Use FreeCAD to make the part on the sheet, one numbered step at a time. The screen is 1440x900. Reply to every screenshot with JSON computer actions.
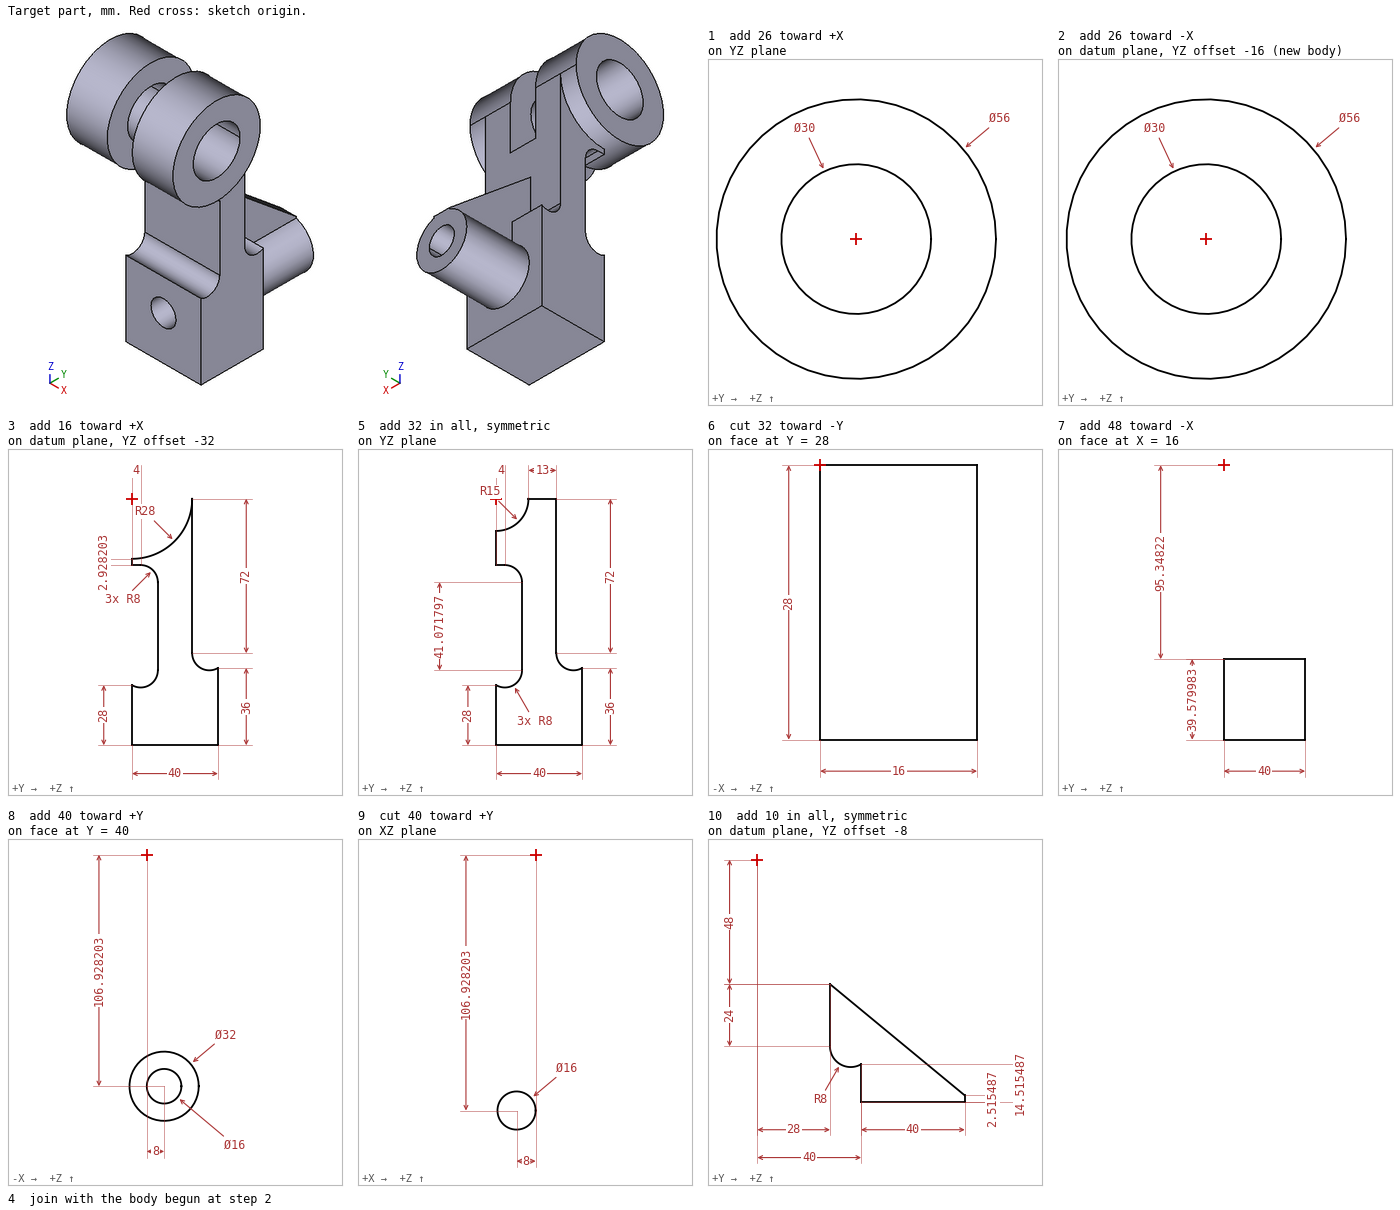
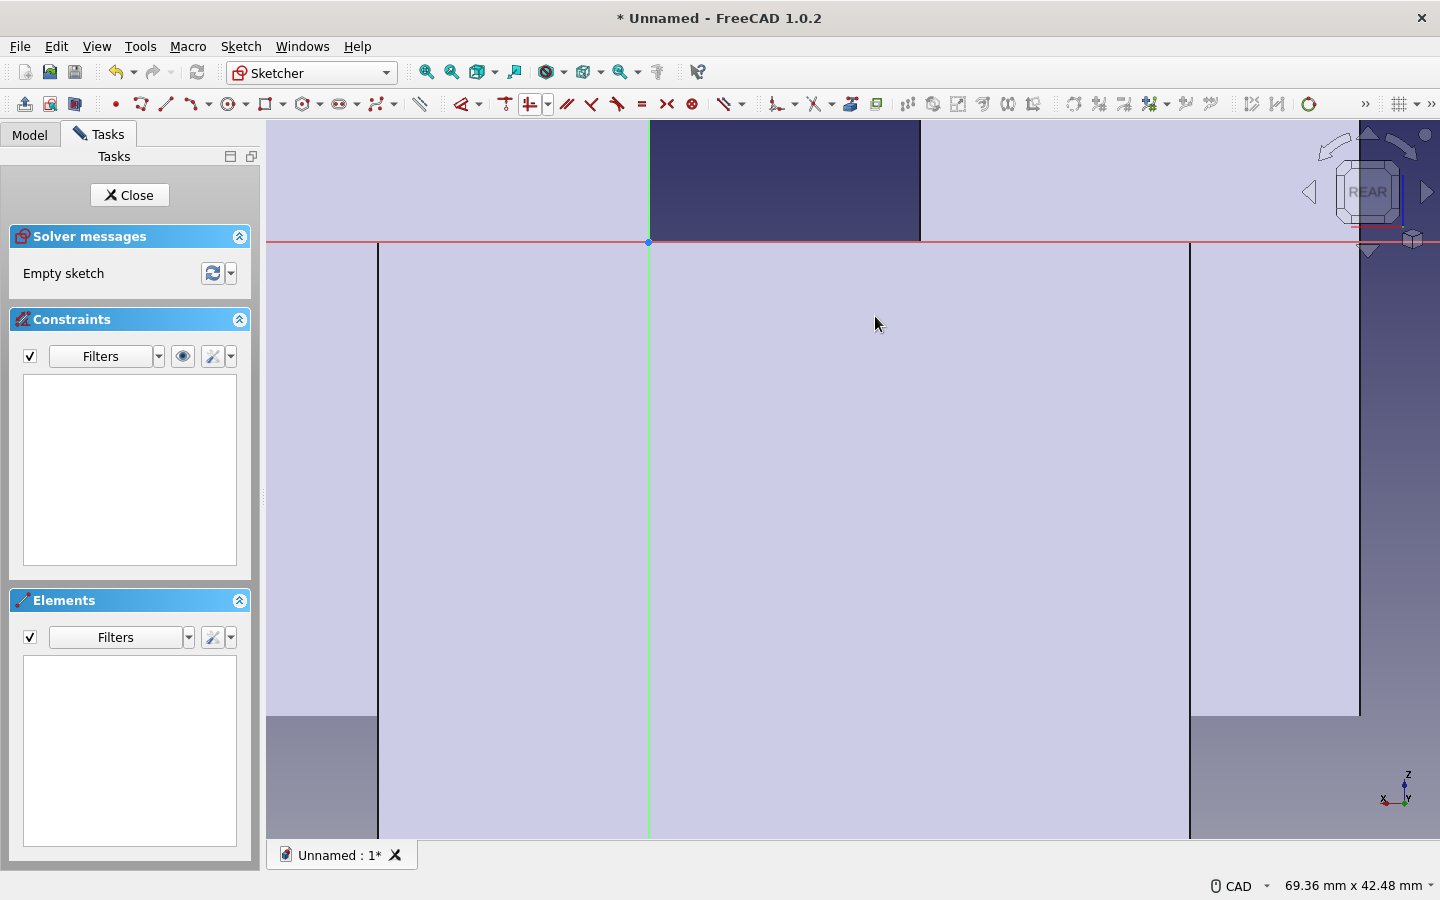
{"action": "key", "text": "g r"}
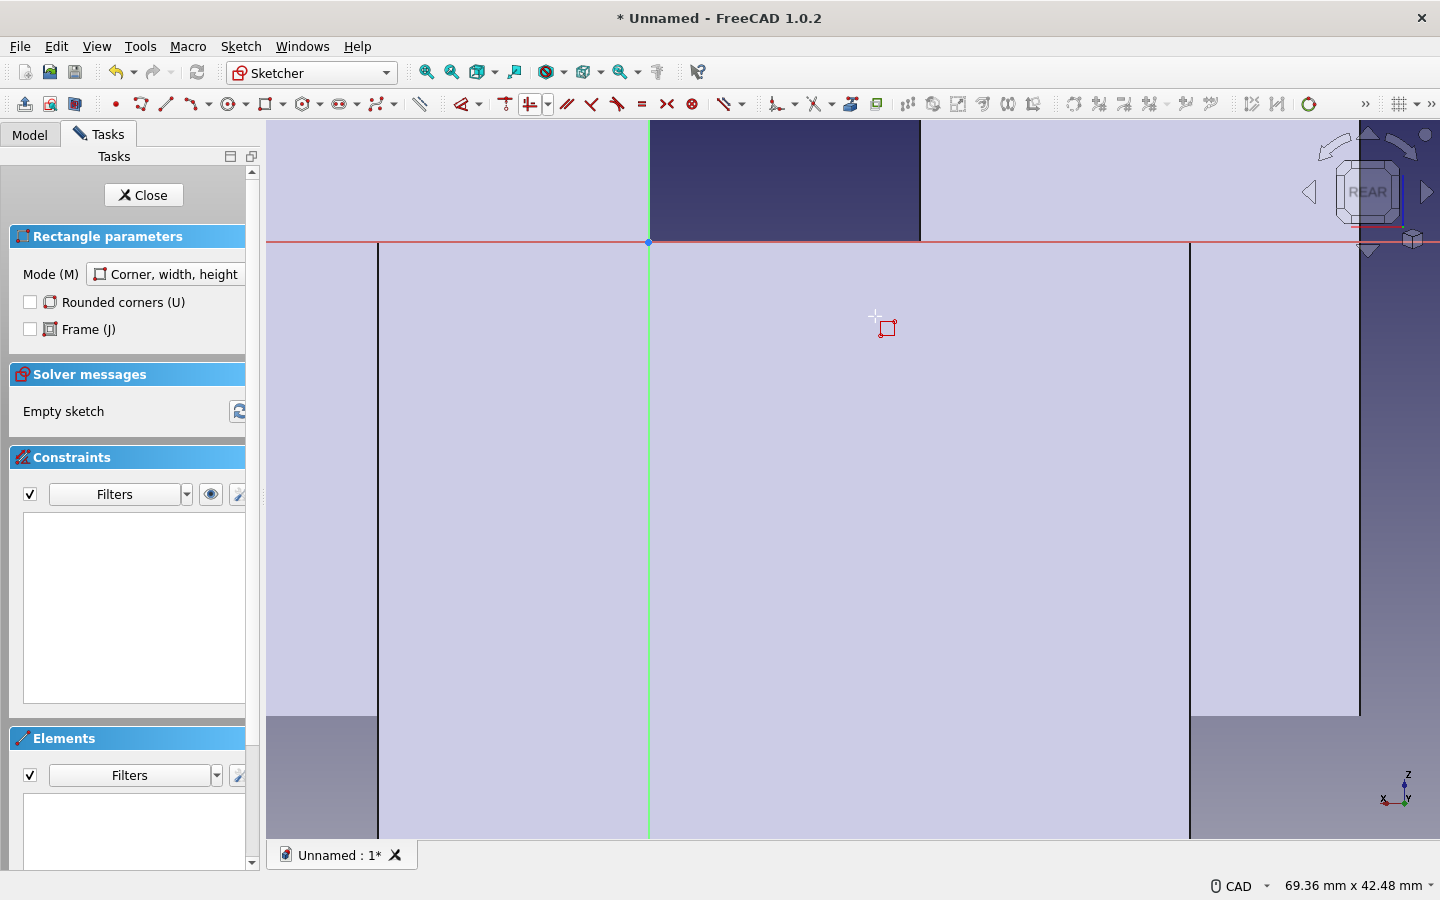
{"action": "left_click", "coordinate": [649, 242]}
{"action": "left_click", "coordinate": [920, 716]}
{"action": "key", "text": "Escape"}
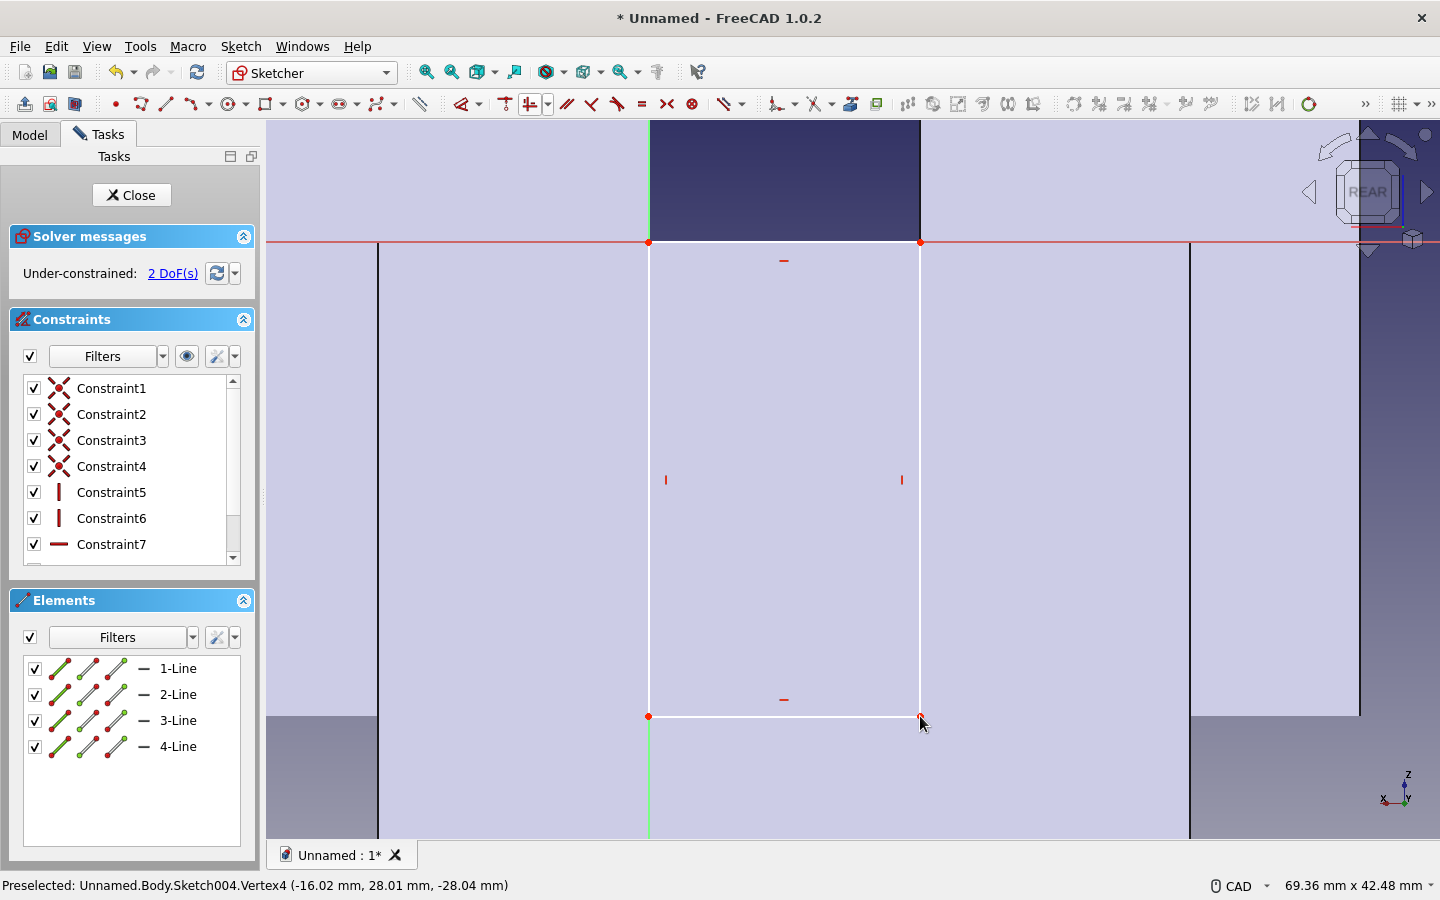
{"action": "left_click", "coordinate": [460, 104]}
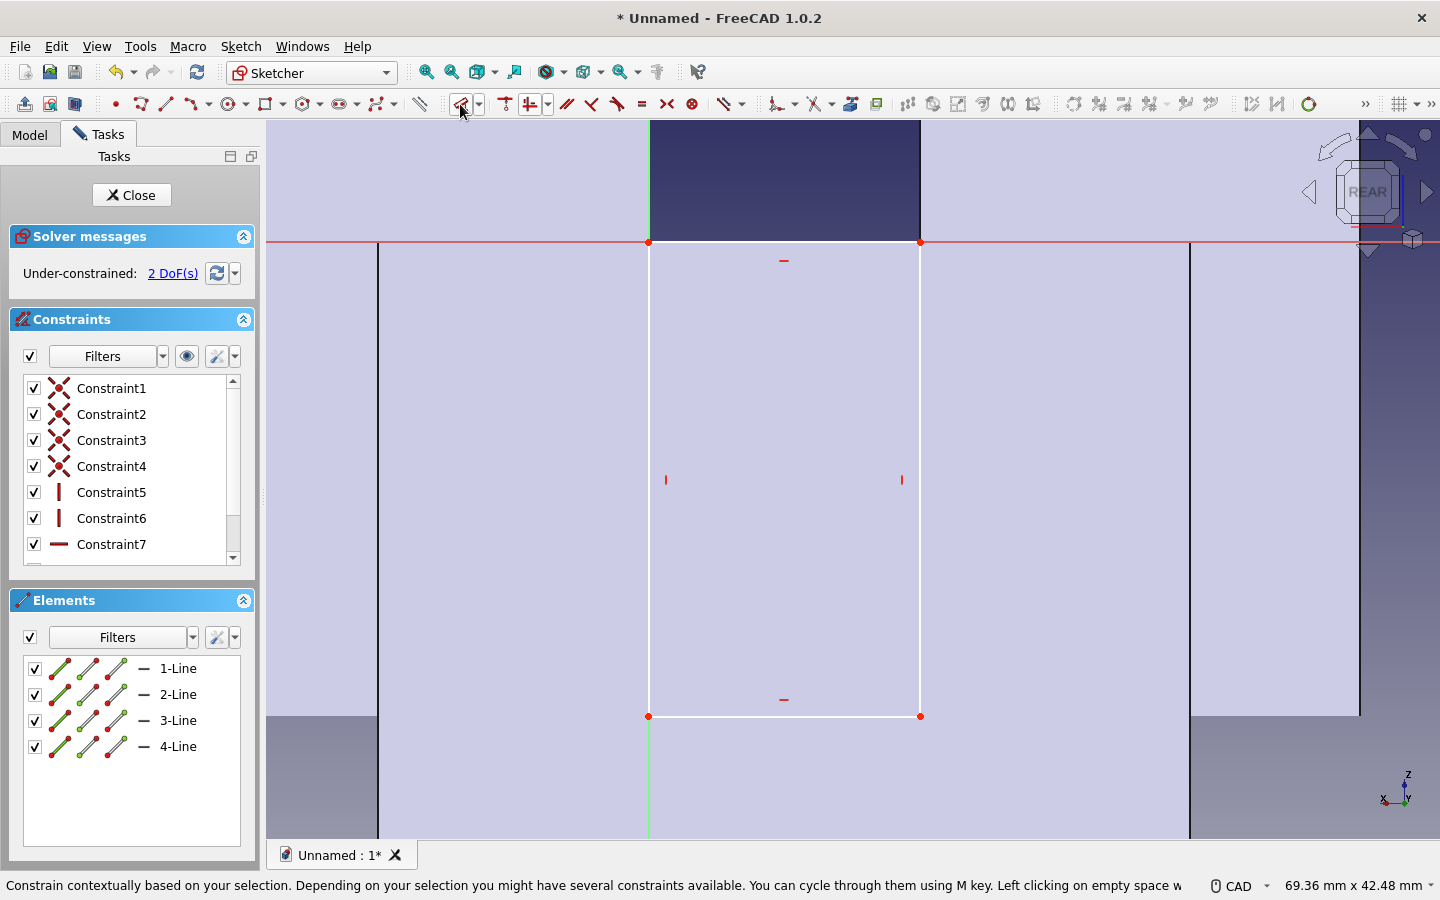
{"action": "left_click", "coordinate": [649, 385]}
{"action": "left_click", "coordinate": [615, 480]}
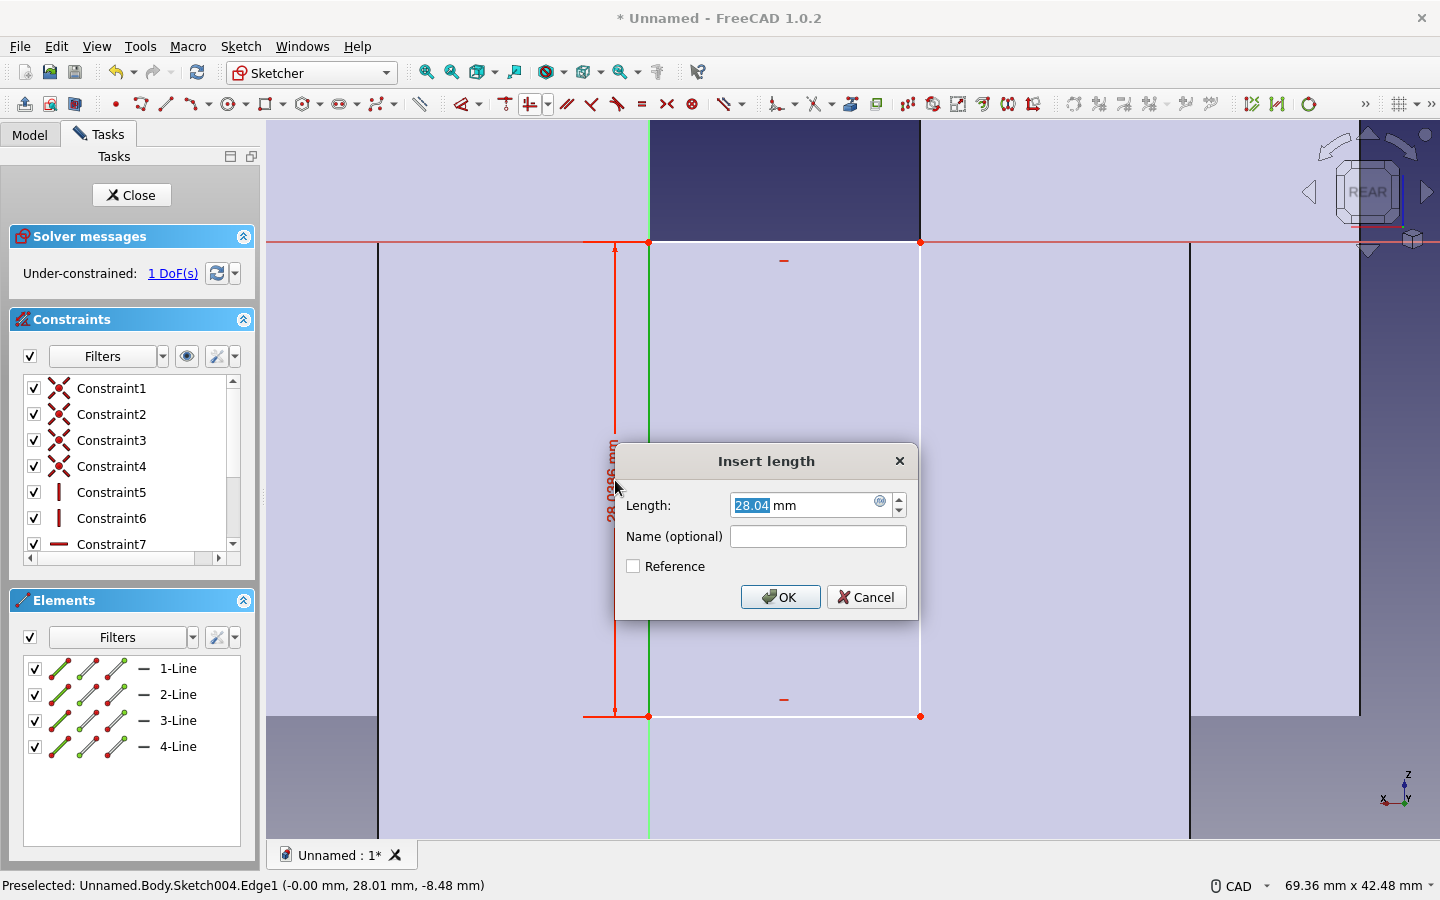
{"action": "type", "text": "28"}
{"action": "key", "text": "Return"}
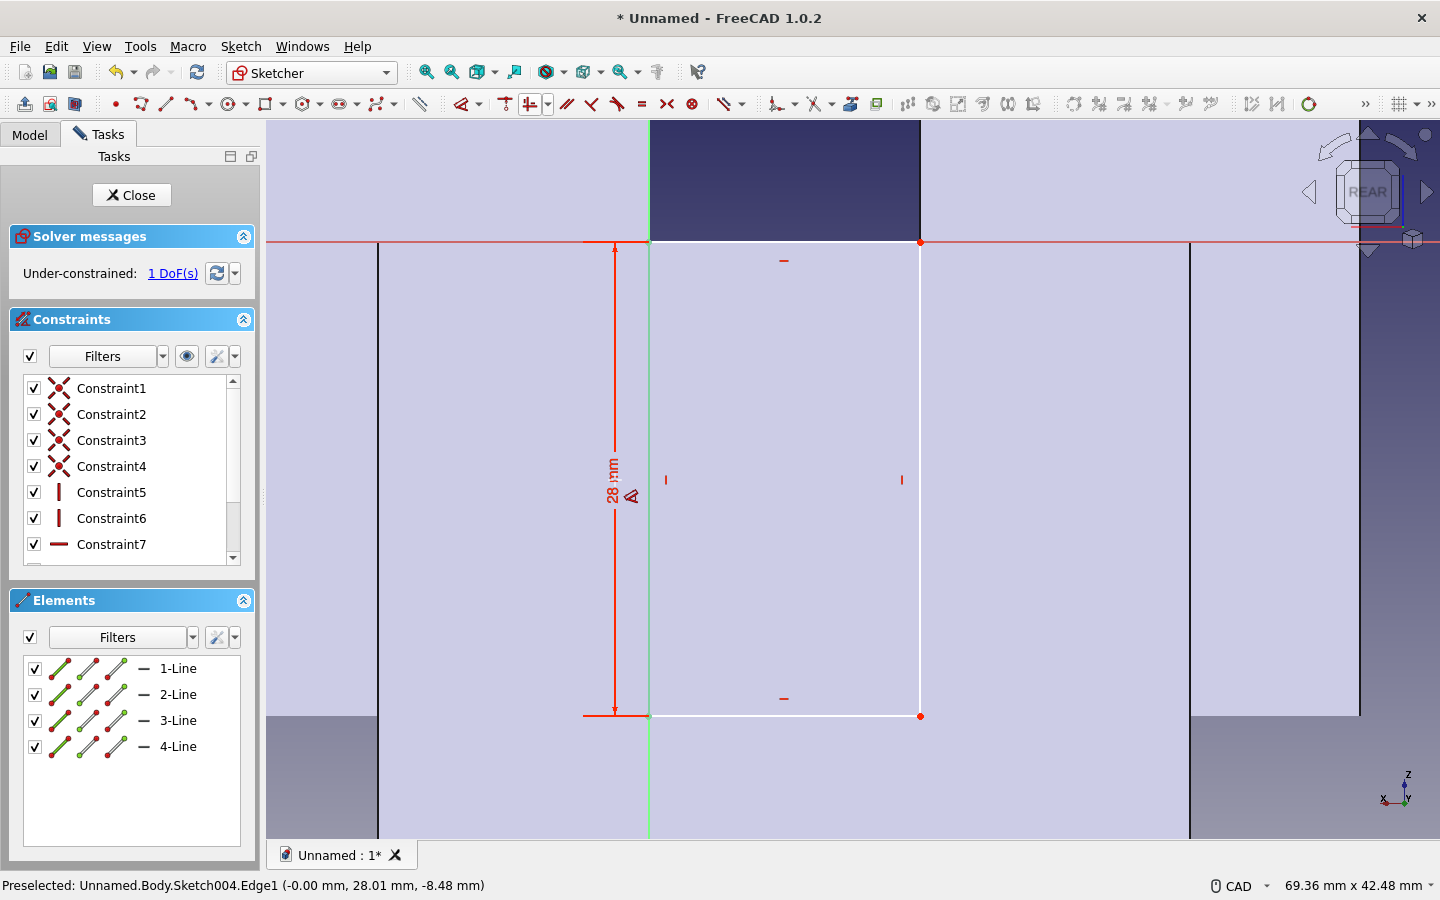
{"action": "left_click", "coordinate": [730, 716]}
{"action": "left_click", "coordinate": [784, 750]}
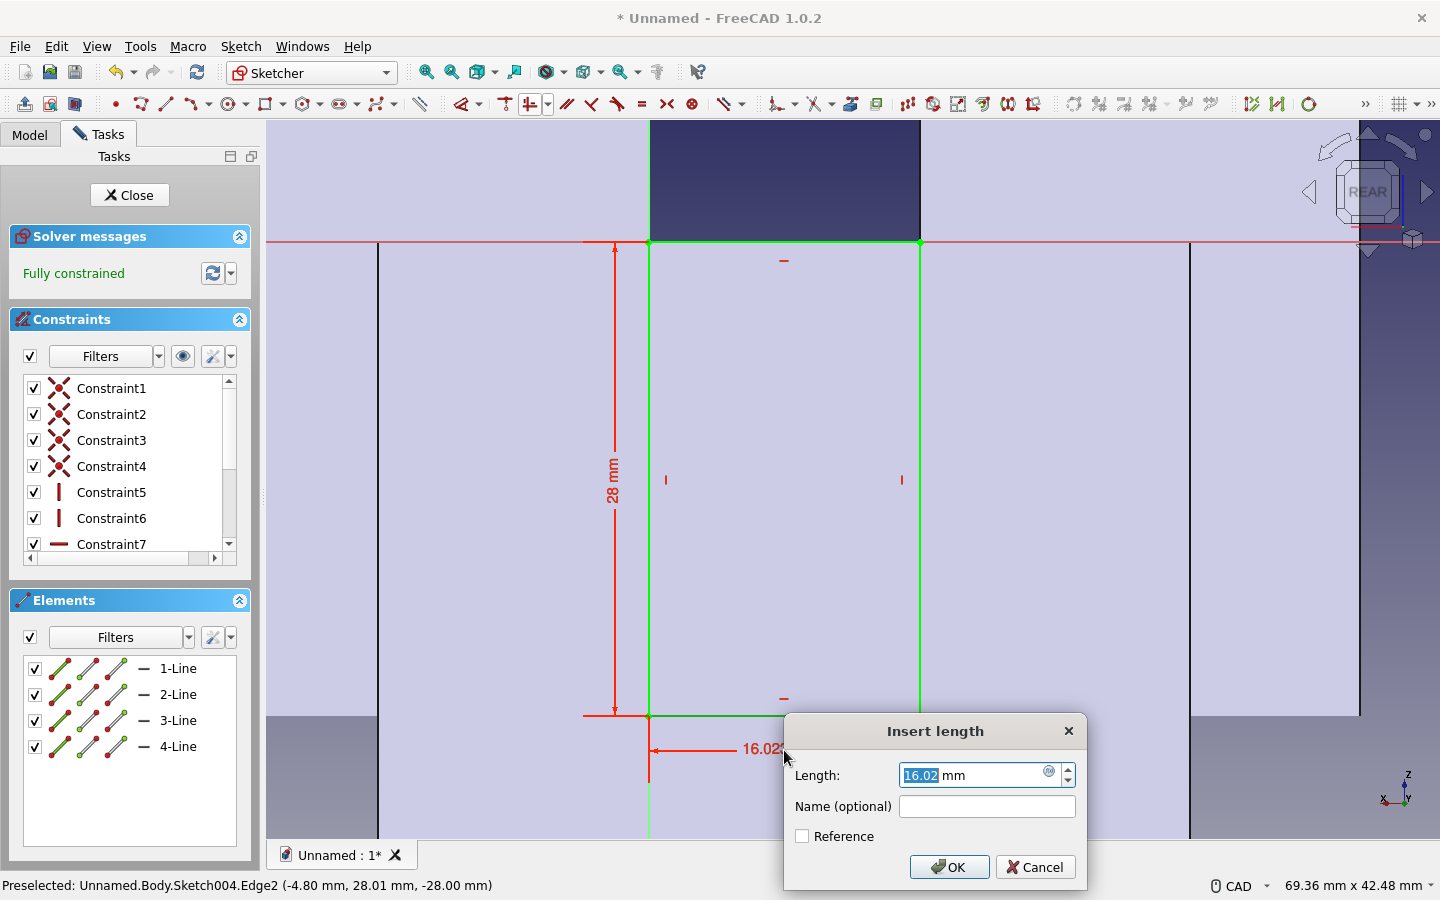
{"action": "type", "text": "16"}
{"action": "key", "text": "Return"}
{"action": "key", "text": "Escape"}